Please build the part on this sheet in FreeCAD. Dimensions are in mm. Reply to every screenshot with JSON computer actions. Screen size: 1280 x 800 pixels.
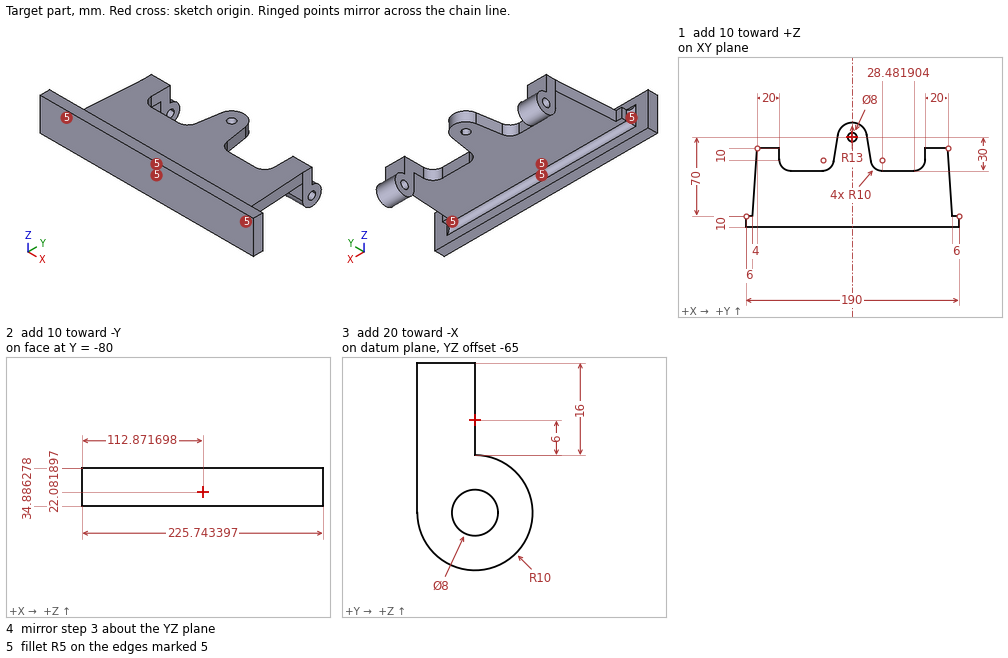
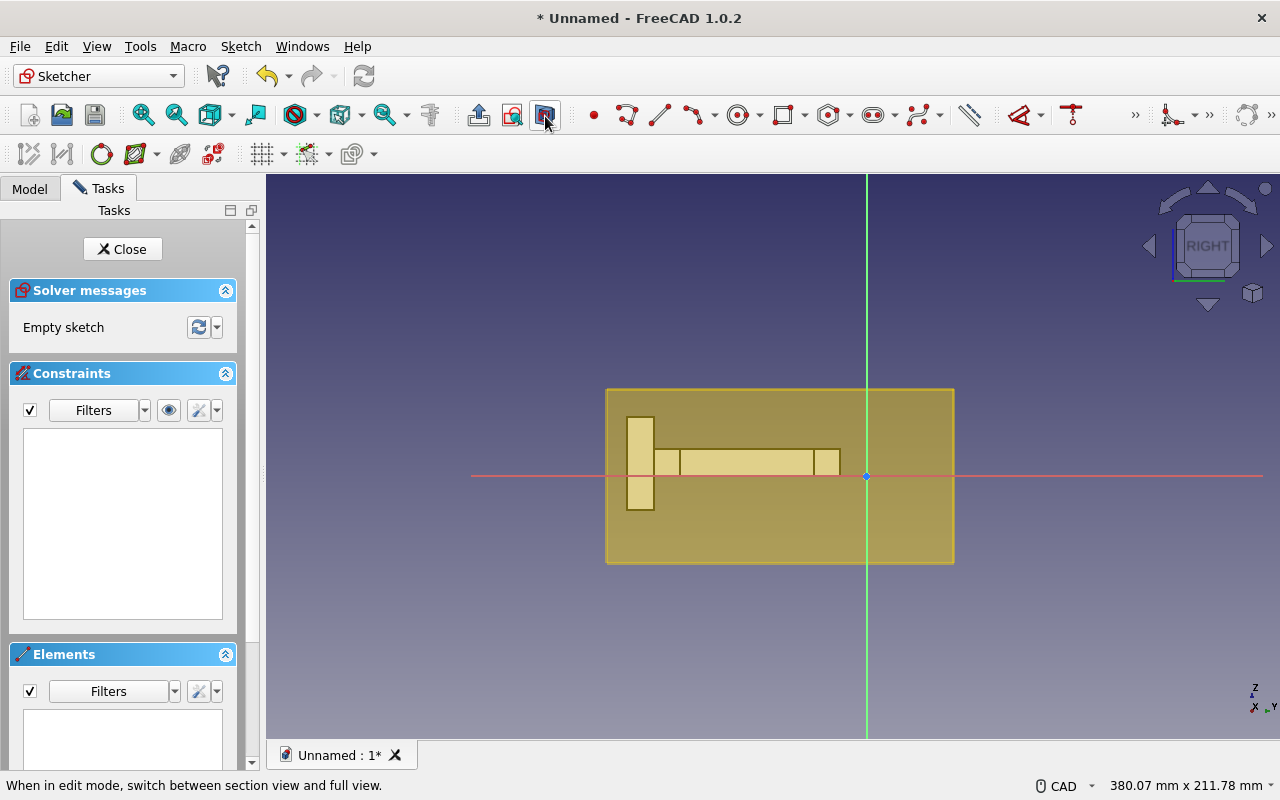
{"action": "scroll", "coordinate": [915, 506], "scroll_direction": "up", "scroll_amount": 7}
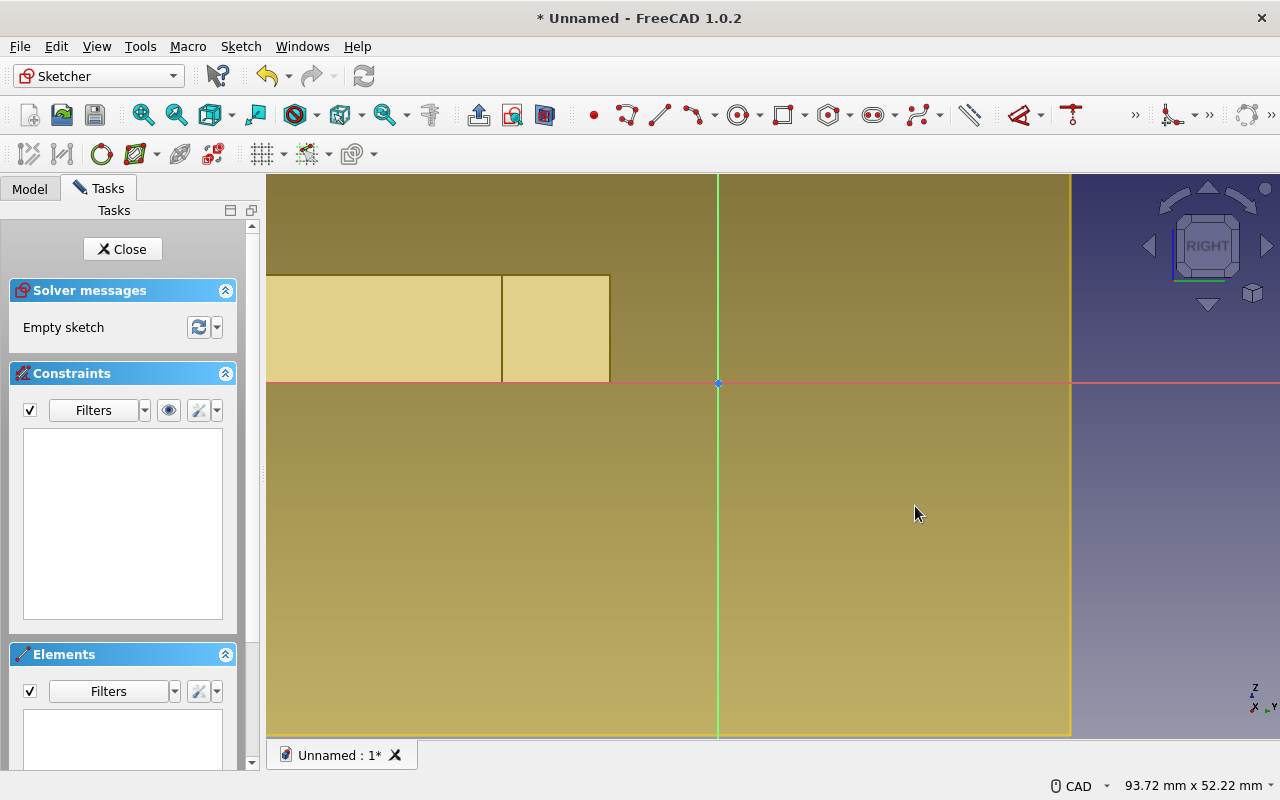
{"action": "left_click", "coordinate": [627, 116]}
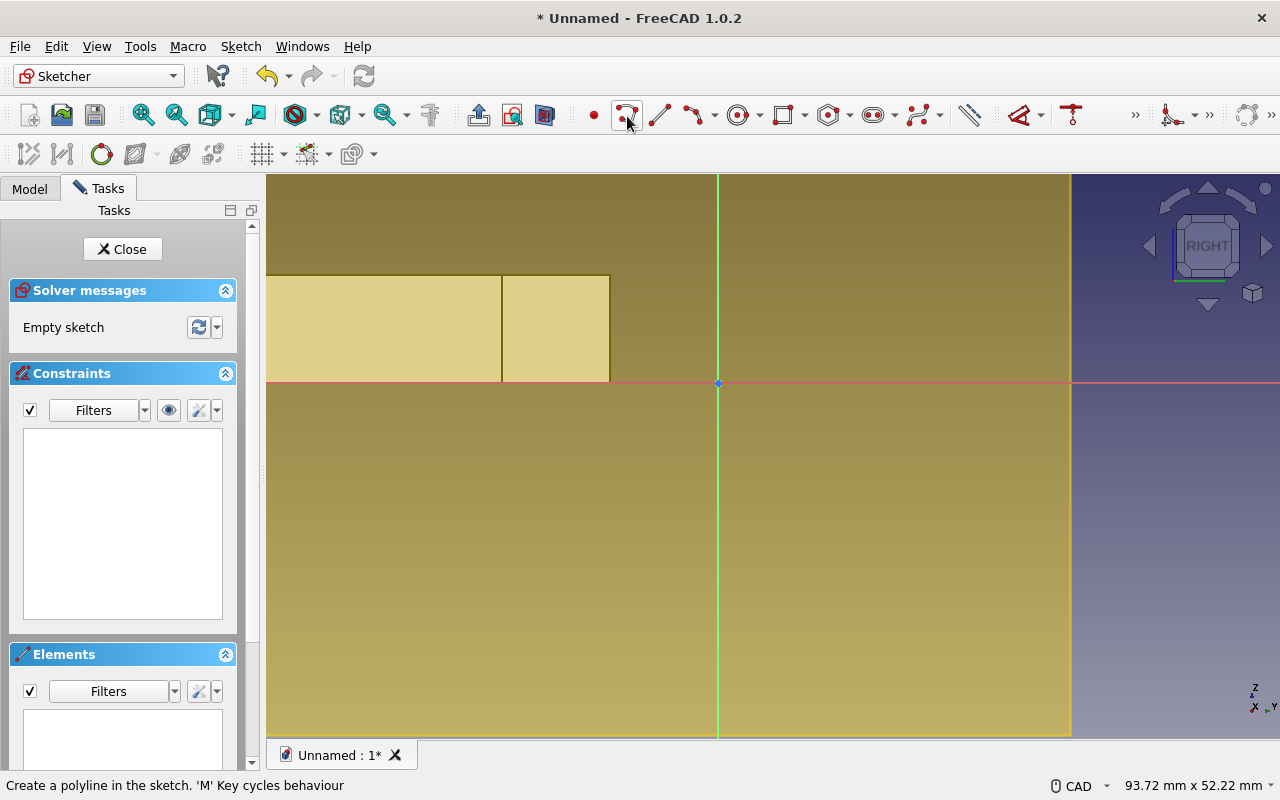
{"action": "left_click", "coordinate": [718, 448]}
{"action": "left_click", "coordinate": [709, 275]}
{"action": "left_click", "coordinate": [610, 275]}
{"action": "left_click", "coordinate": [610, 556]}
{"action": "right_click", "coordinate": [610, 556]}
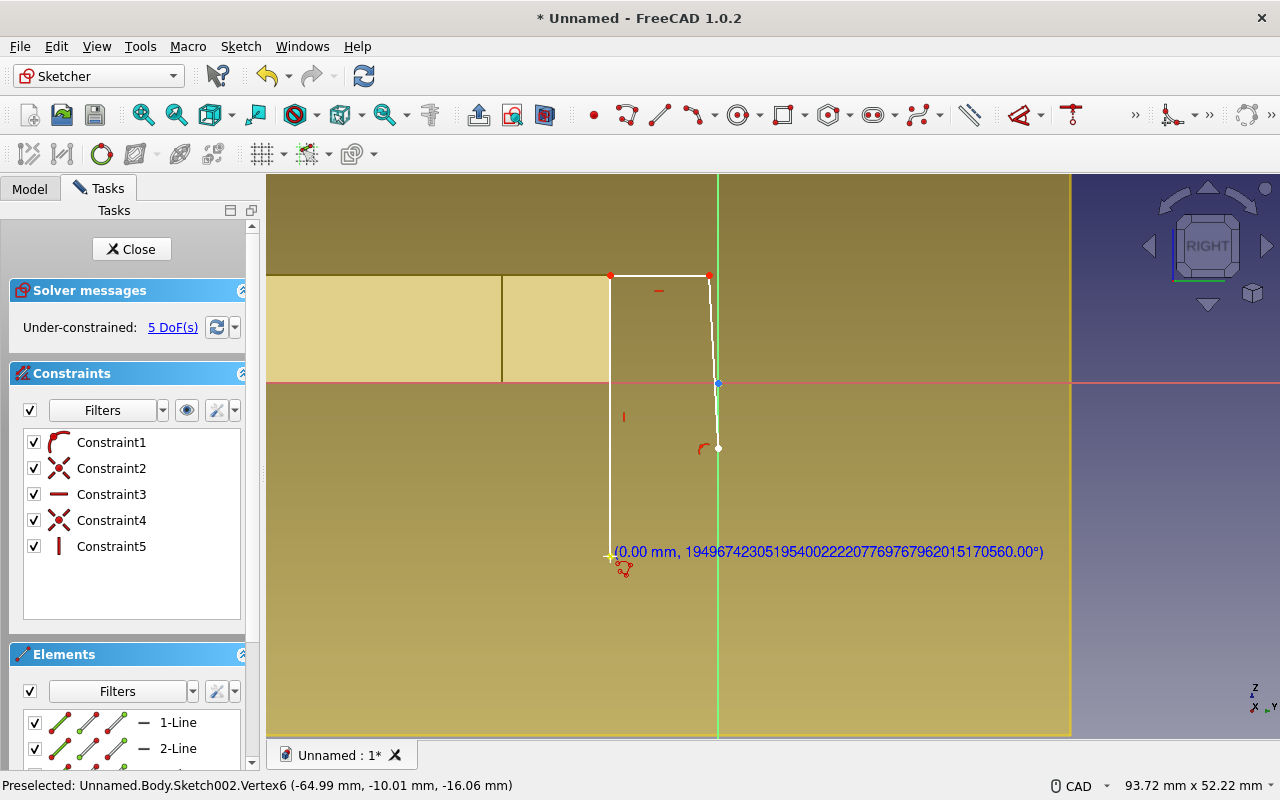
{"action": "key", "text": "g 3 a"}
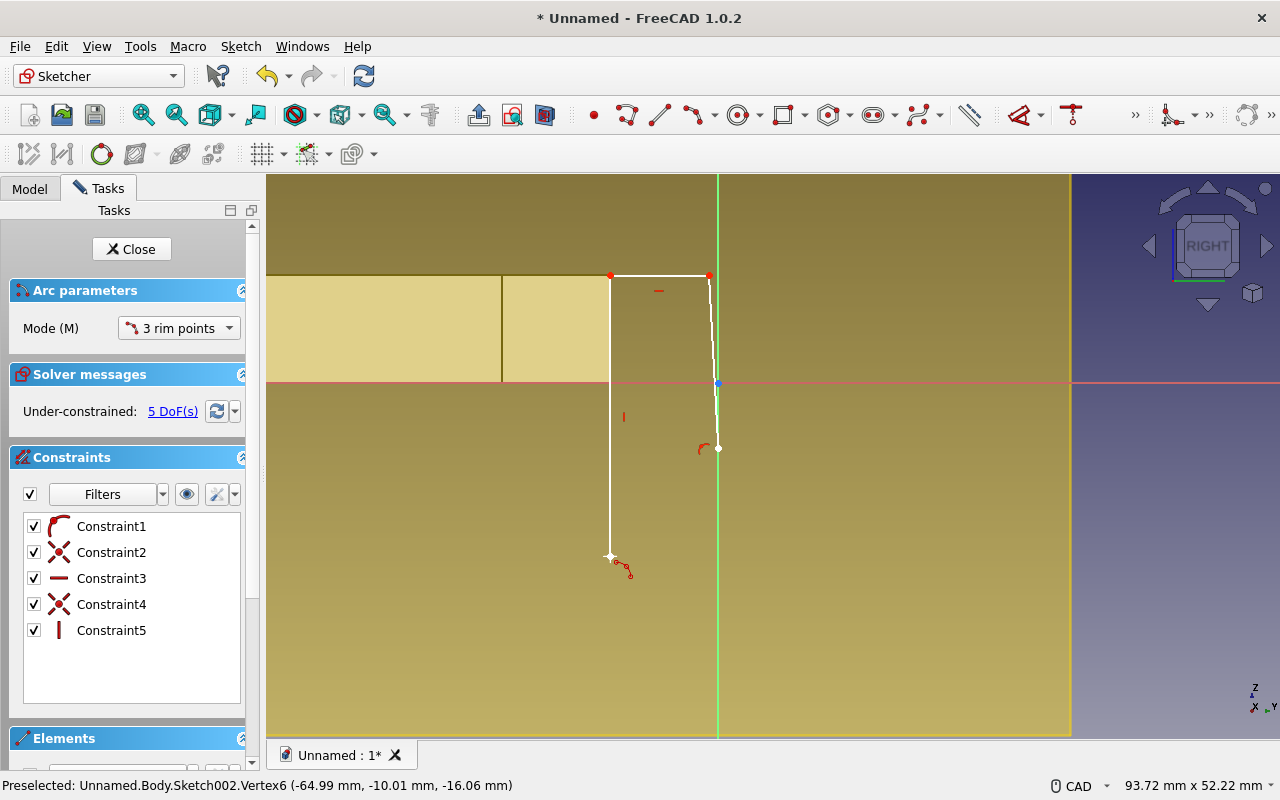
{"action": "left_click", "coordinate": [610, 557]}
{"action": "left_click", "coordinate": [718, 449]}
{"action": "left_click", "coordinate": [795, 633]}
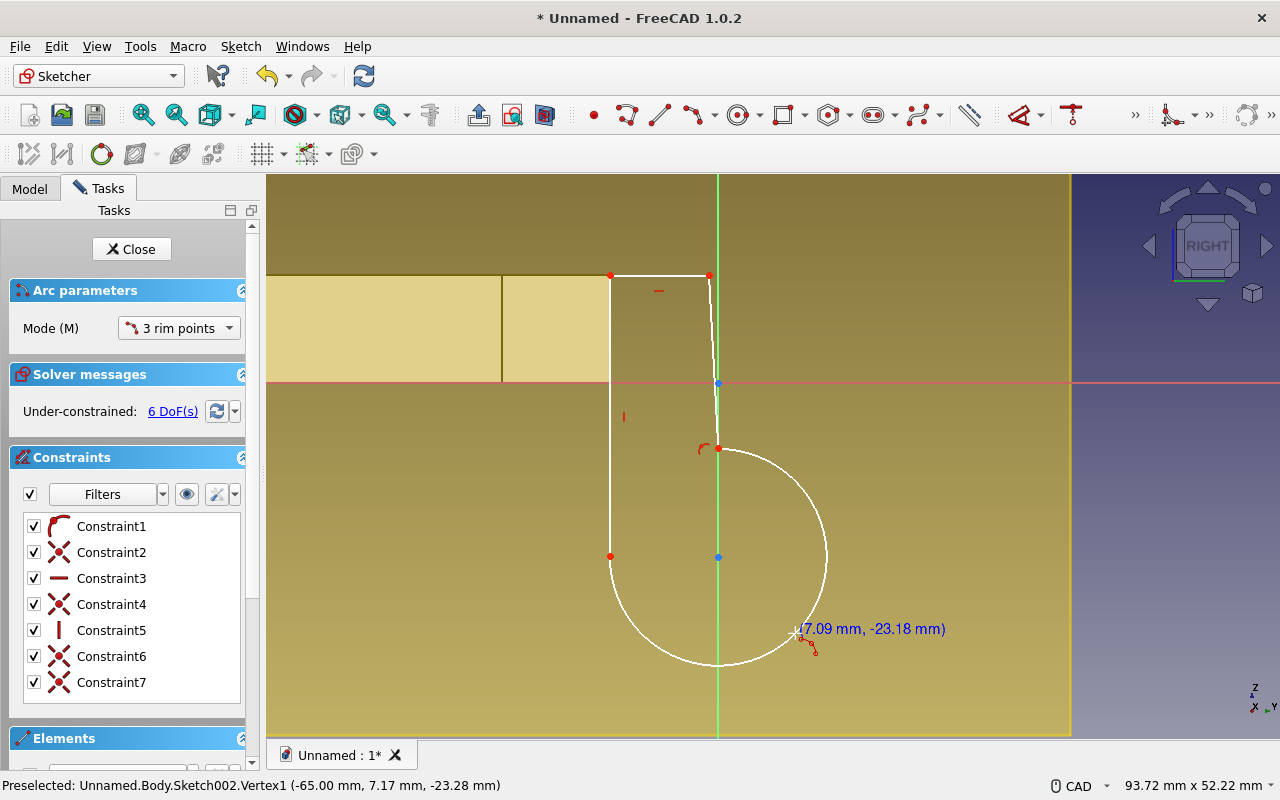
{"action": "key", "text": "g c"}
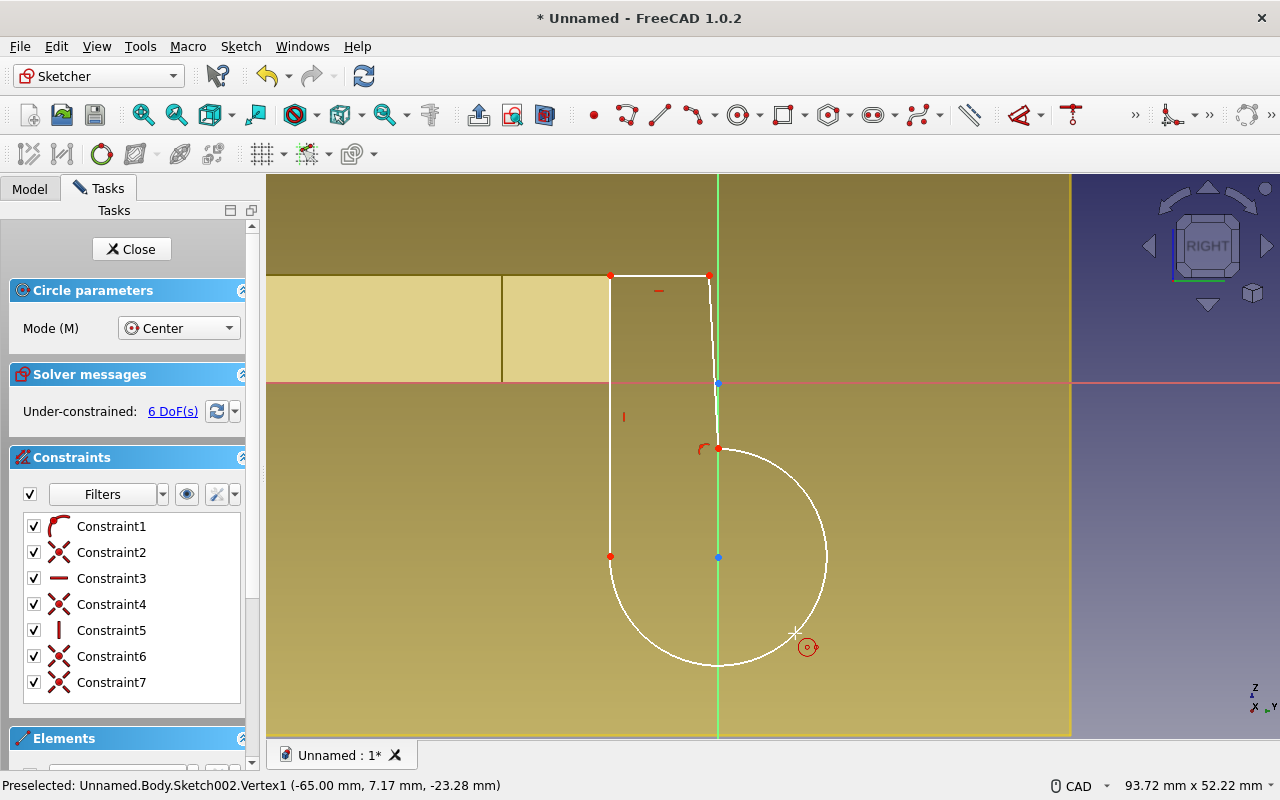
{"action": "left_click", "coordinate": [718, 556]}
{"action": "left_click", "coordinate": [749, 526]}
{"action": "key", "text": "Escape"}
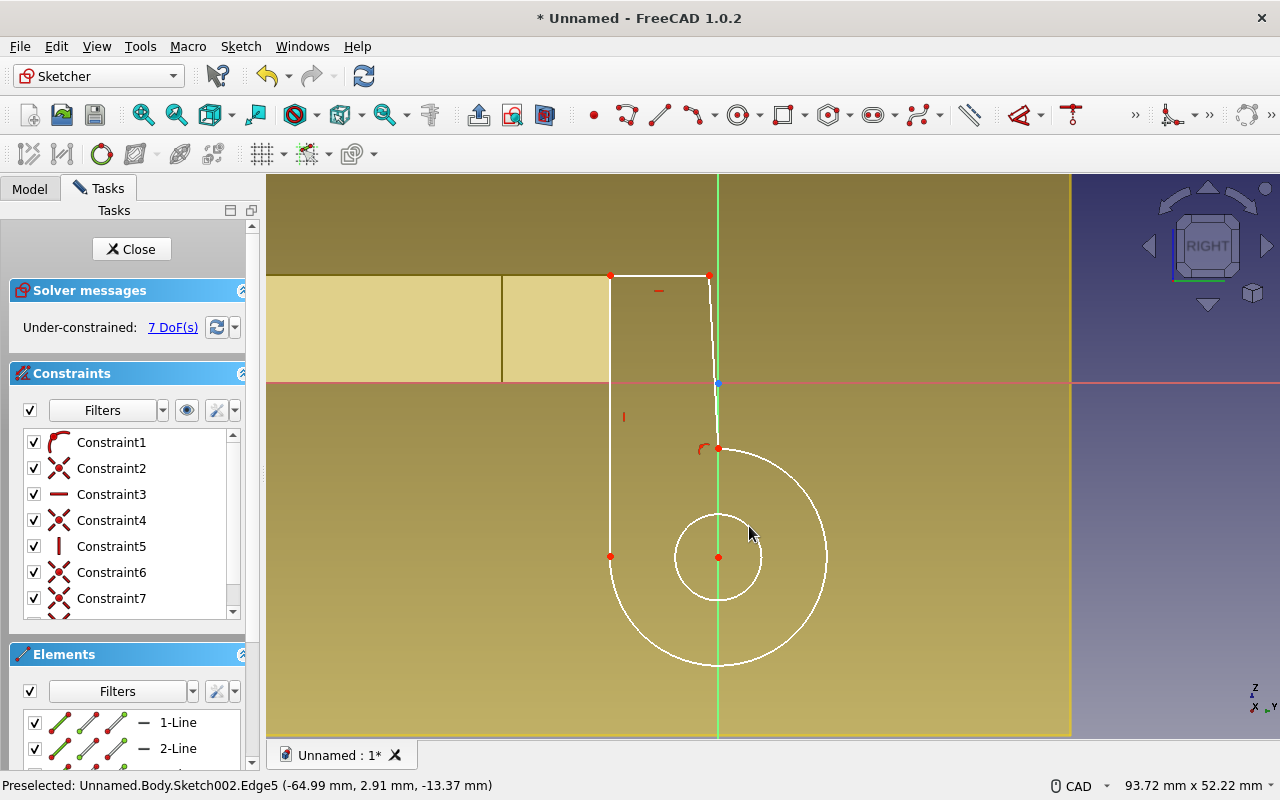
{"action": "left_click", "coordinate": [610, 360]}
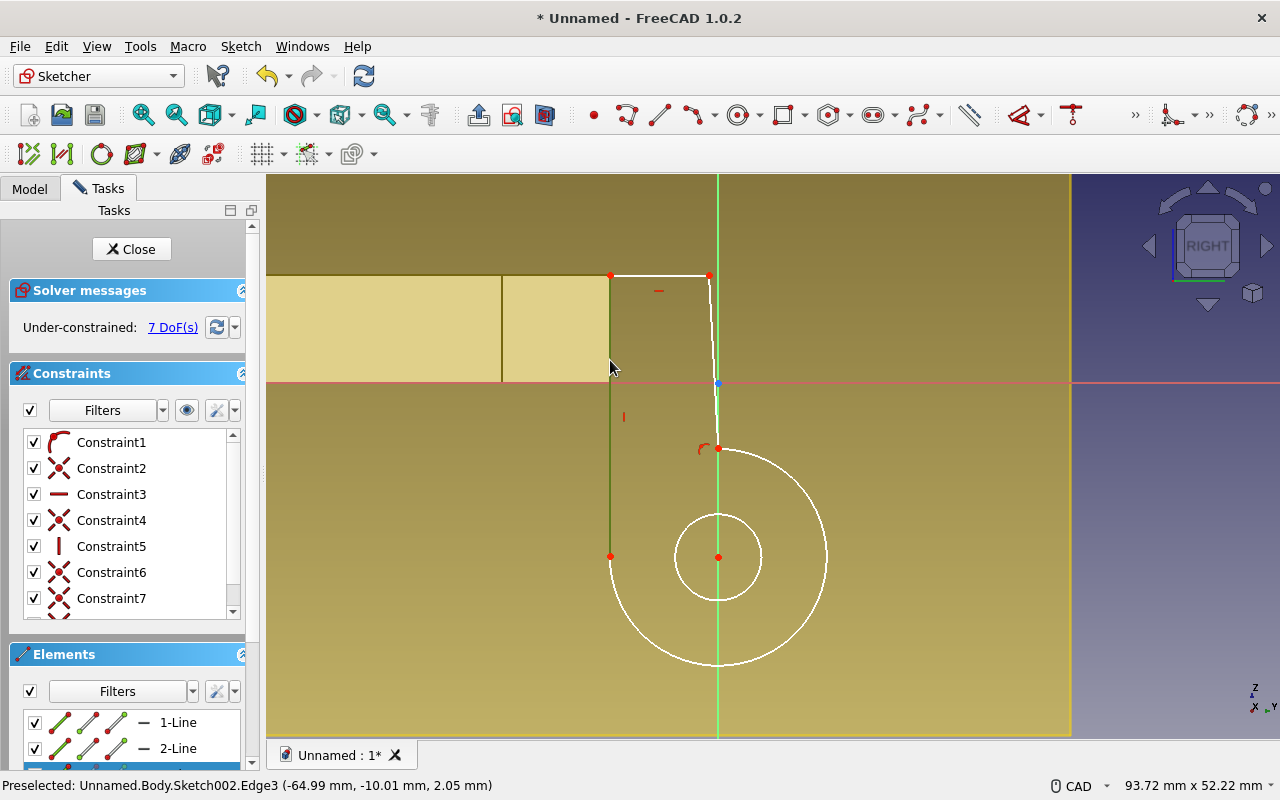
{"action": "left_click", "coordinate": [701, 664]}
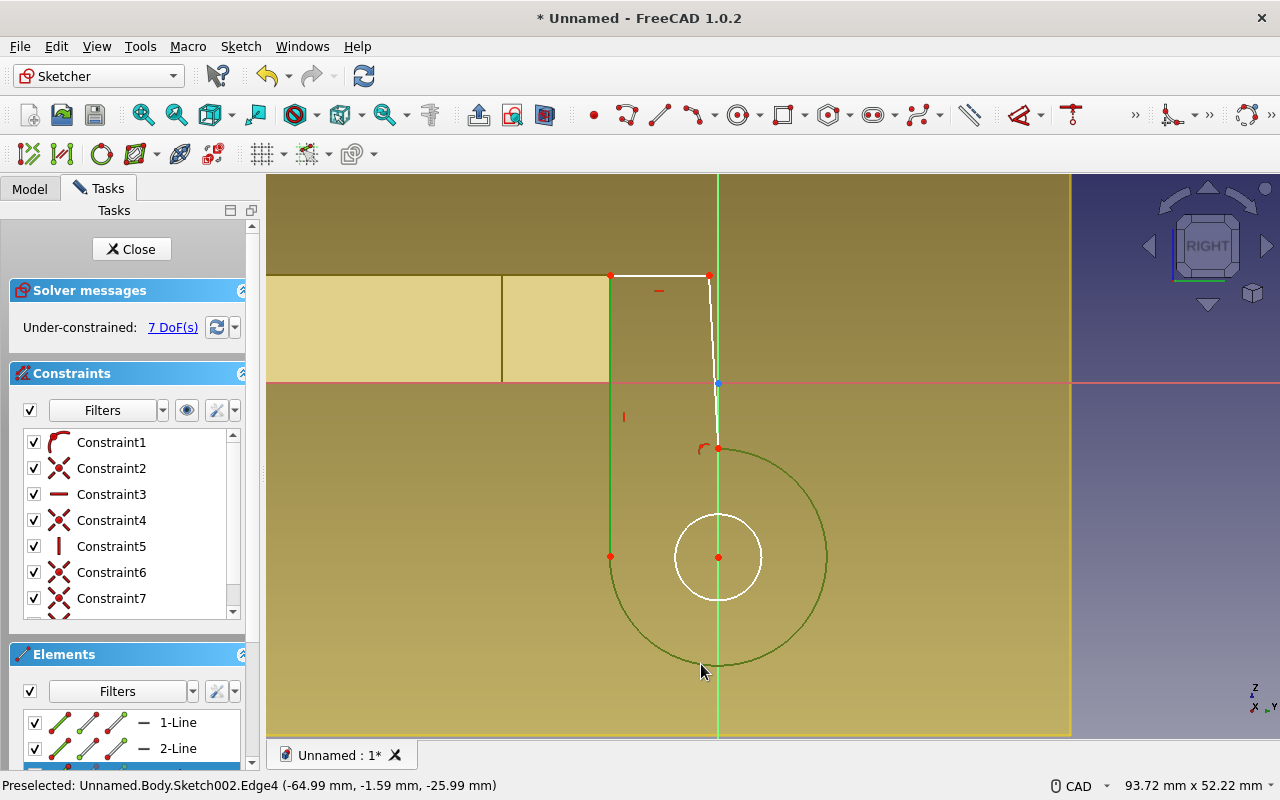
{"action": "key", "text": "t"}